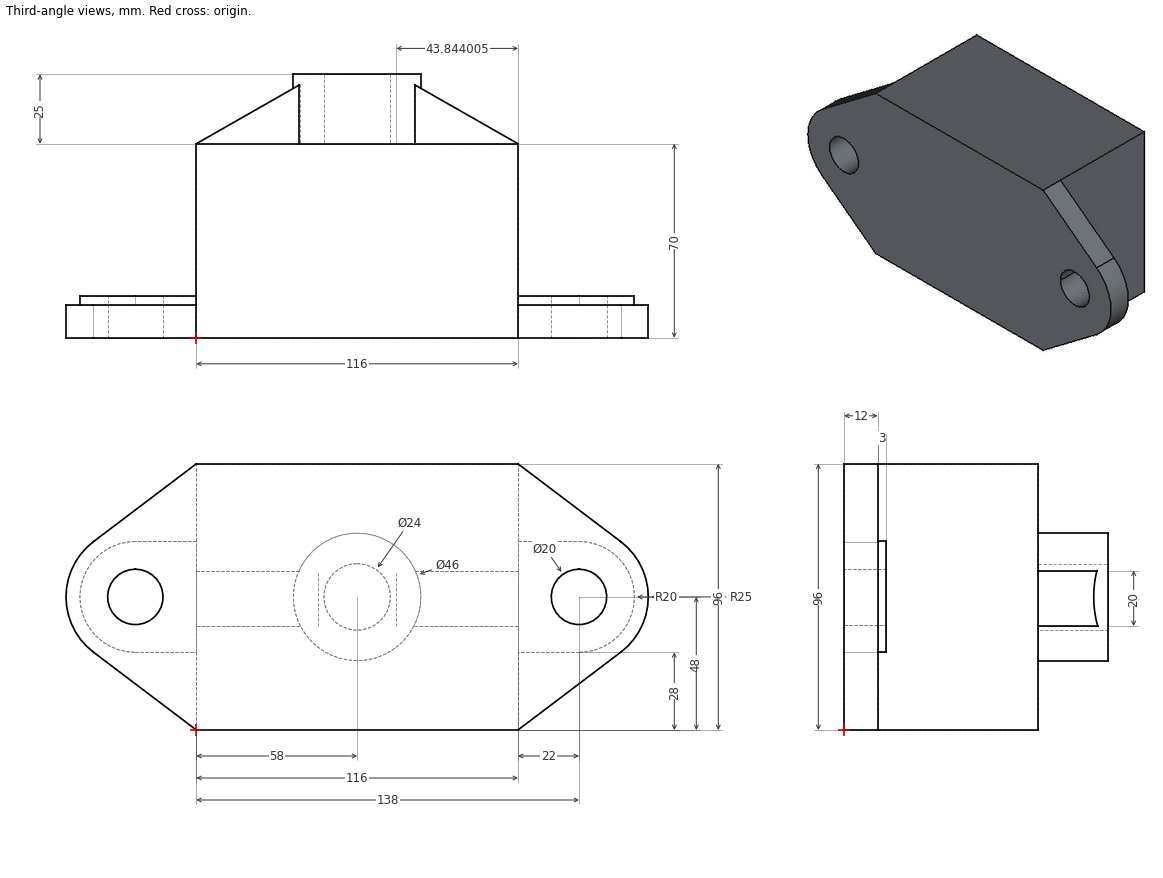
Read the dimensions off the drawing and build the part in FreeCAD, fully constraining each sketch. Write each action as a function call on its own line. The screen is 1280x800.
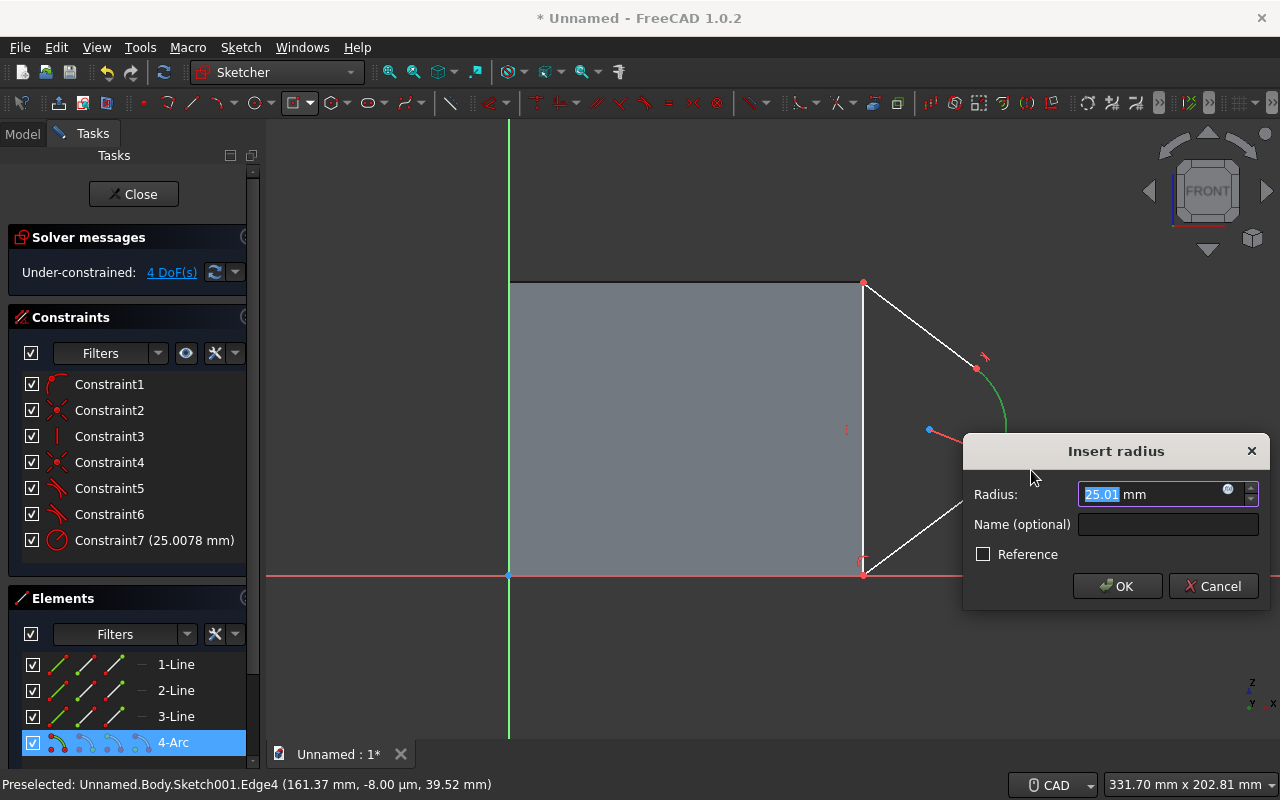
text(25)
key(Return)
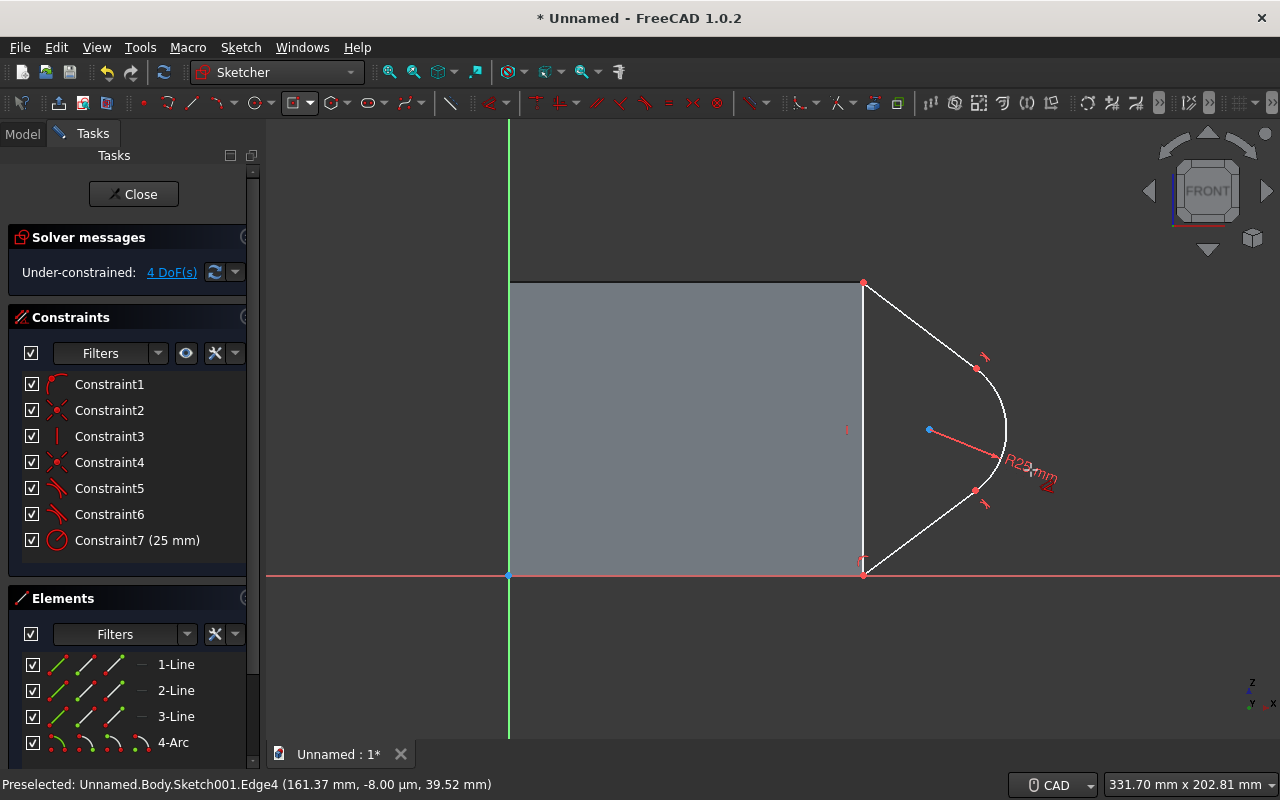
click(863, 488)
click(897, 429)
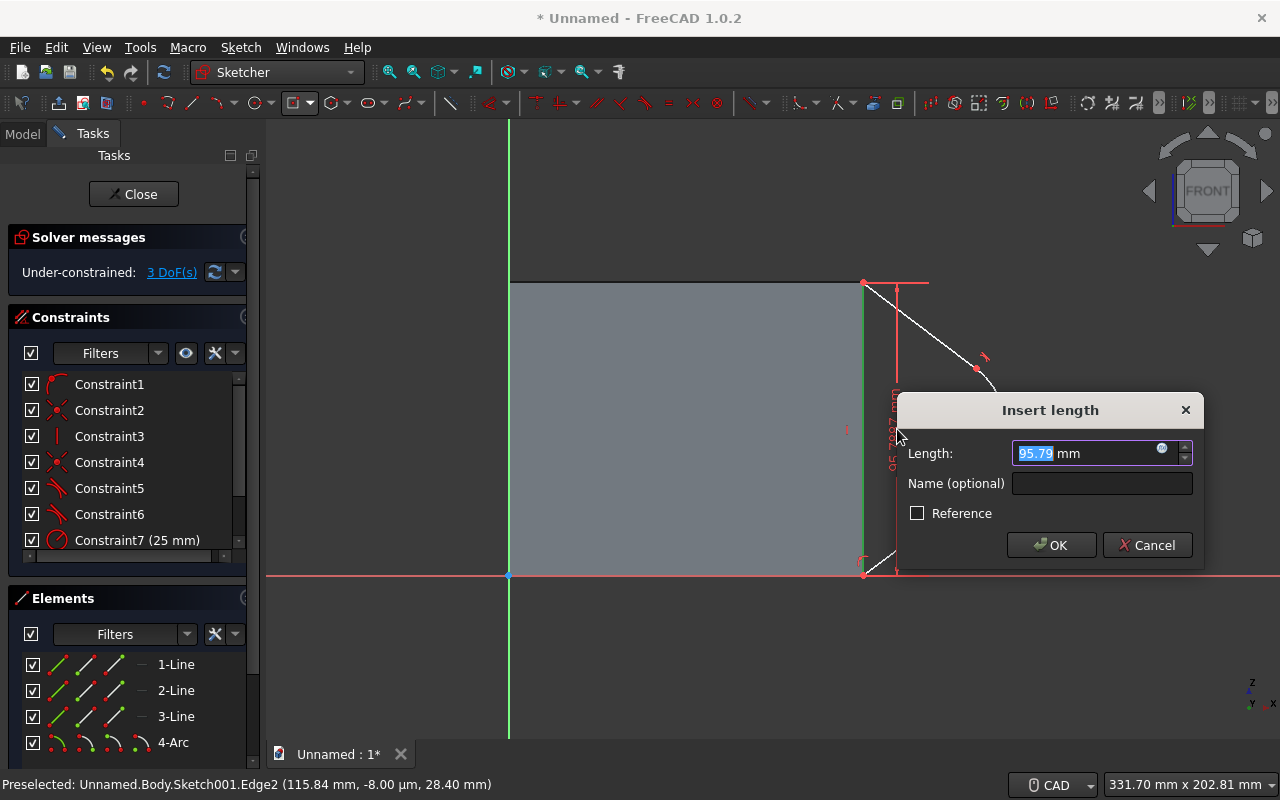
text(96)
key(Return)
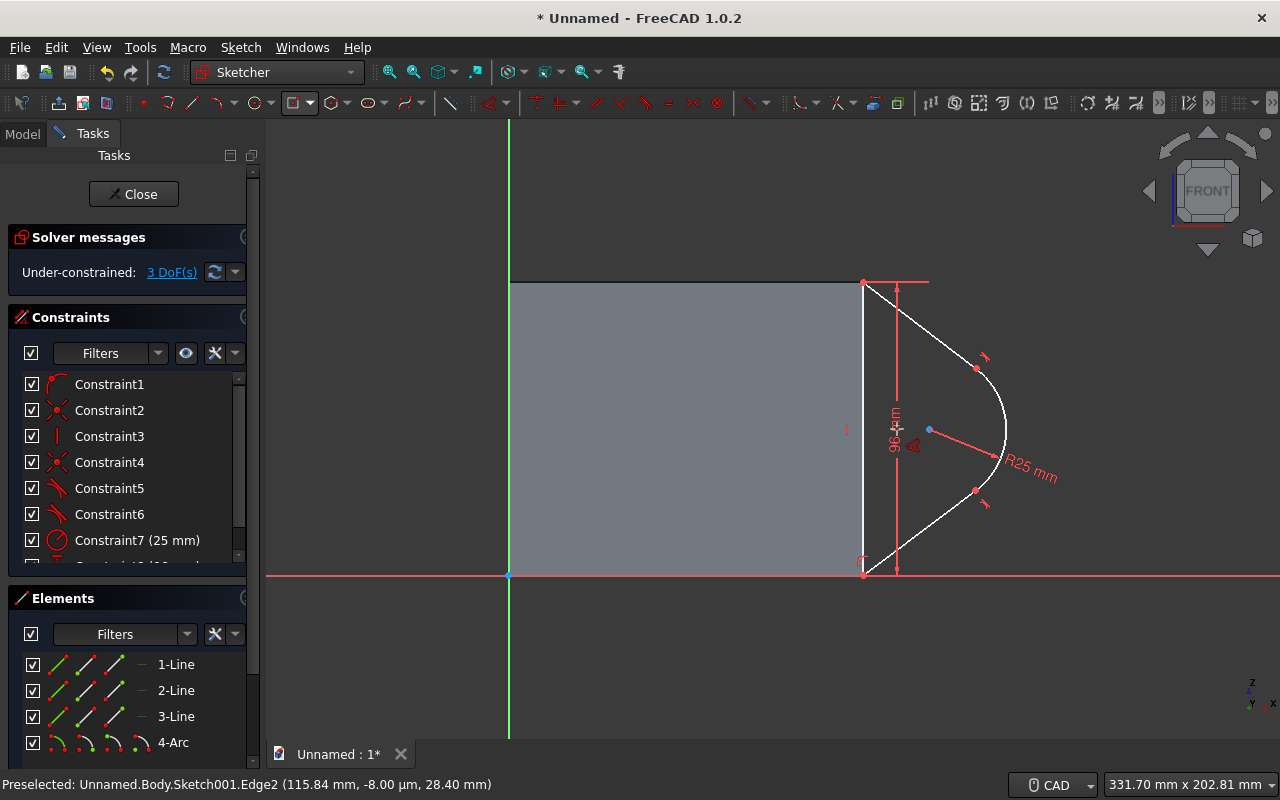
click(930, 430)
click(475, 503)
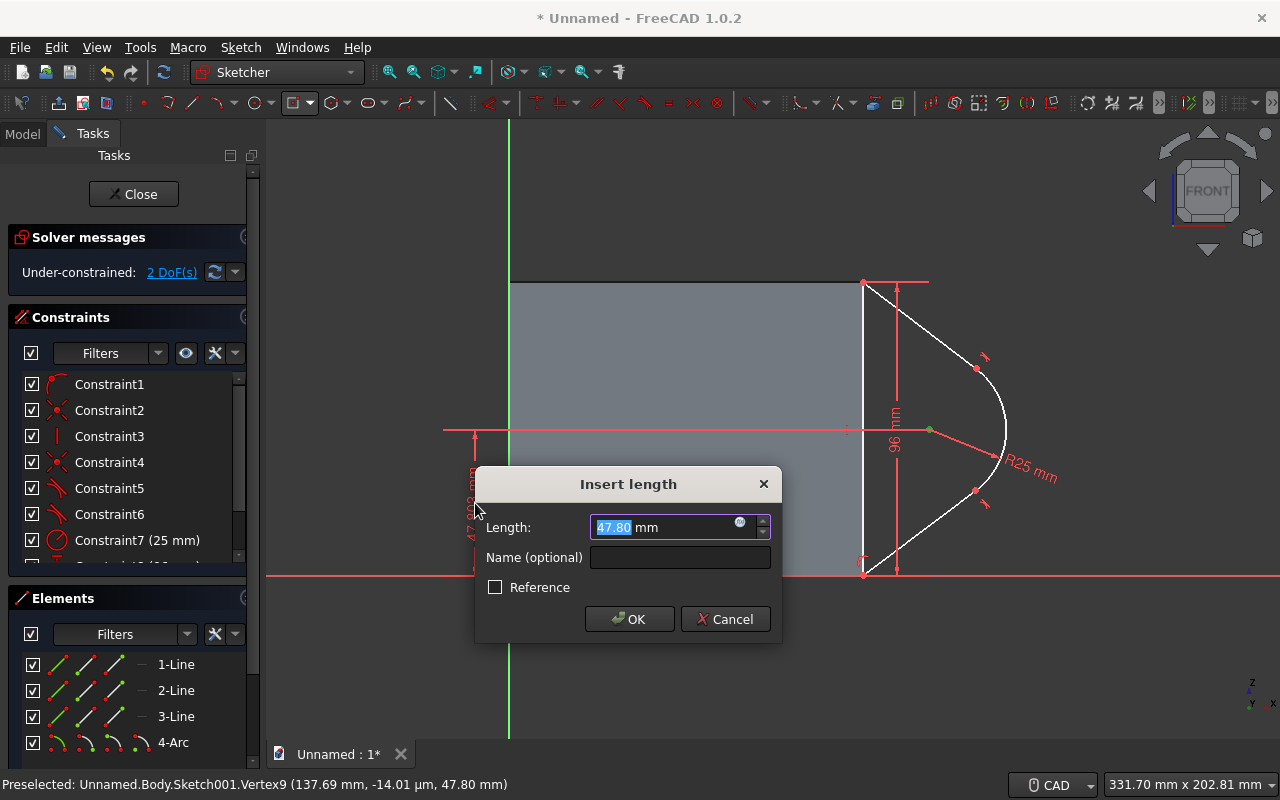
text(48)
key(Return)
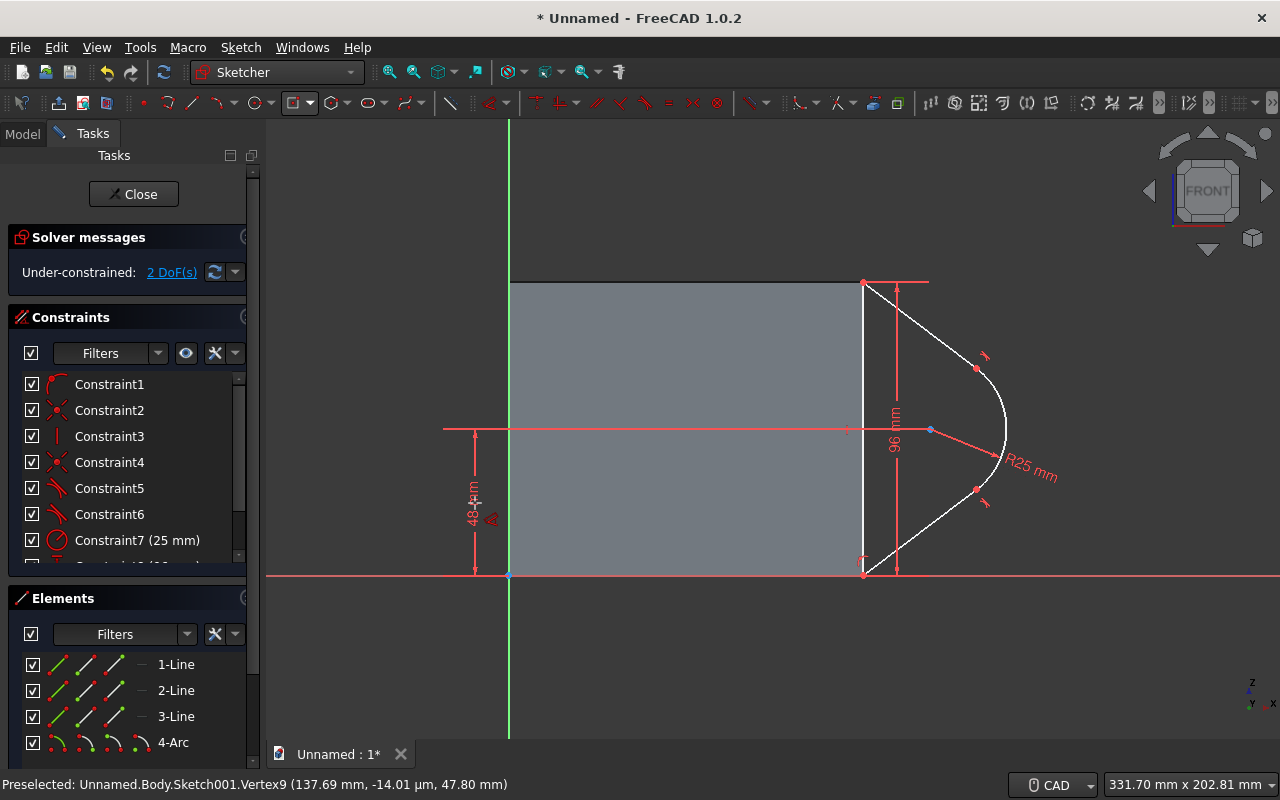
click(863, 576)
click(686, 610)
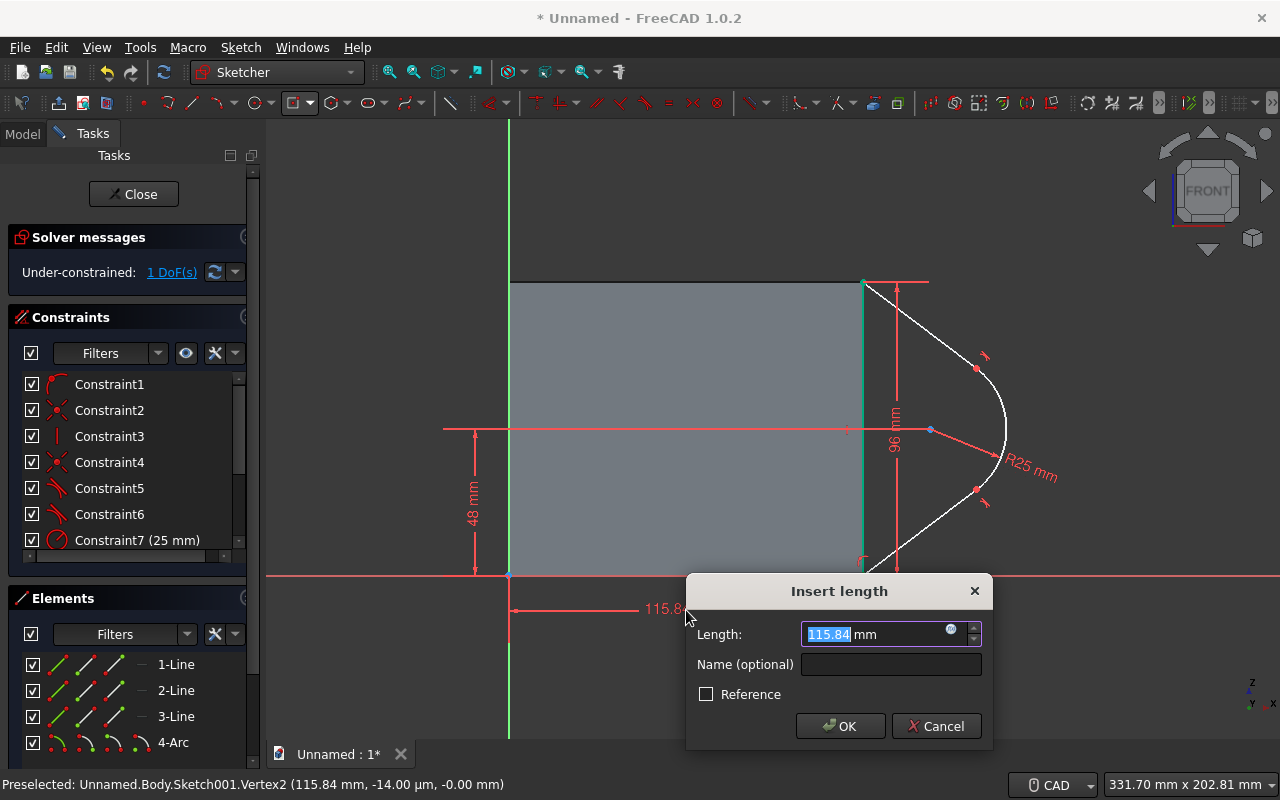
text(116)
key(Return)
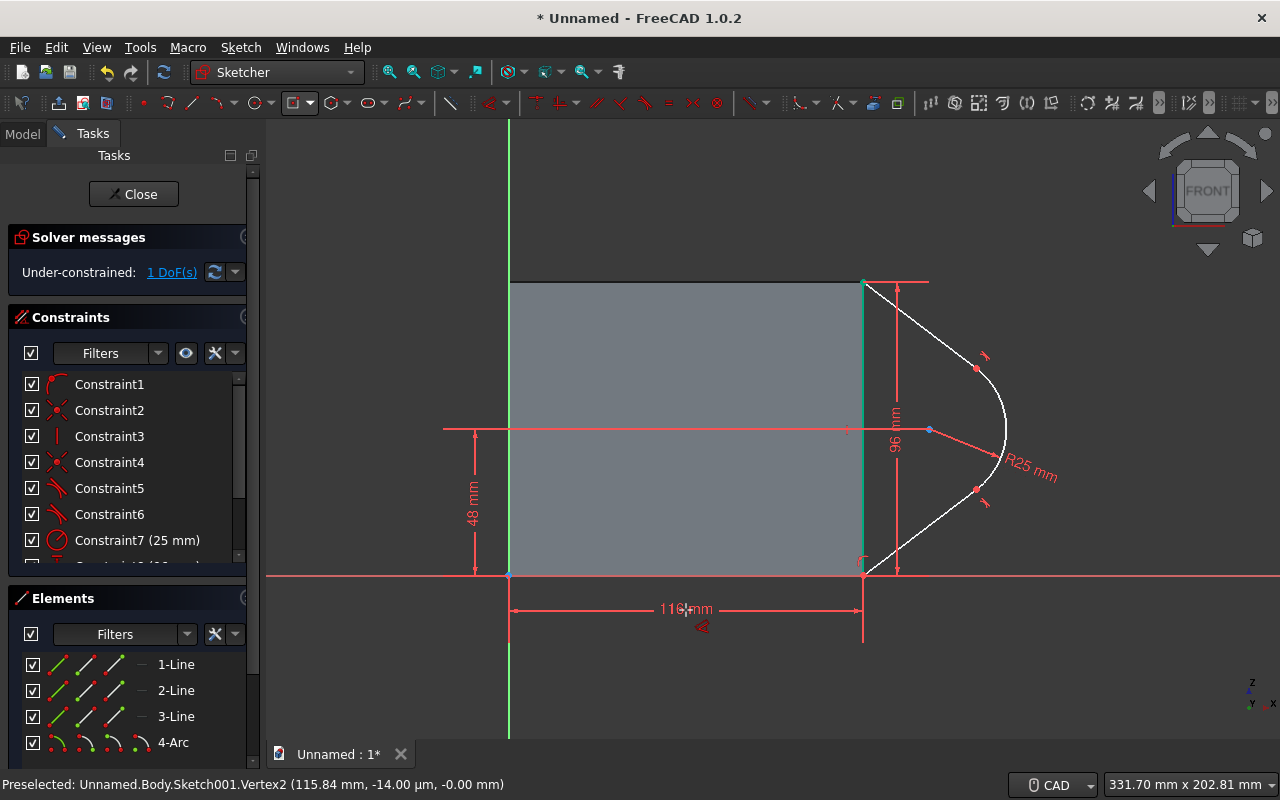
click(930, 429)
click(816, 610)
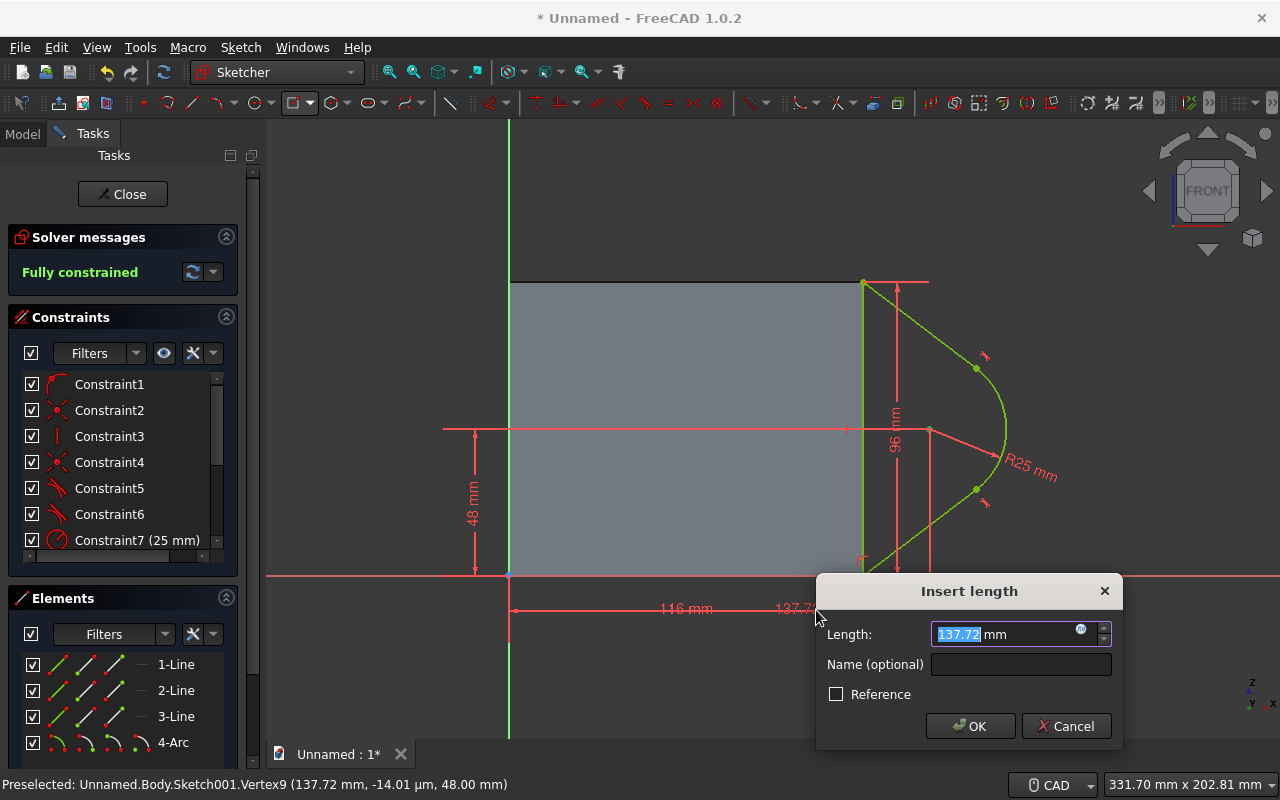
text(138)
key(Return)
key(Escape)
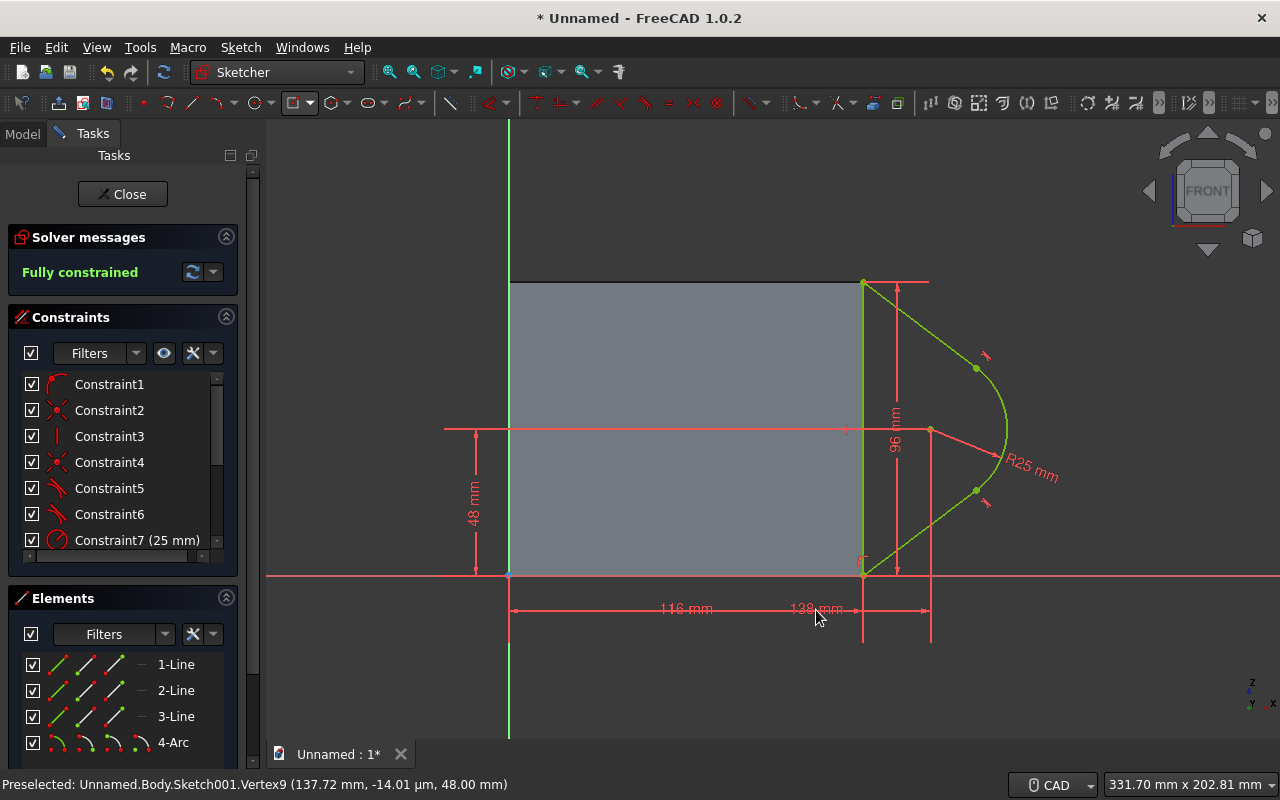
click(123, 194)